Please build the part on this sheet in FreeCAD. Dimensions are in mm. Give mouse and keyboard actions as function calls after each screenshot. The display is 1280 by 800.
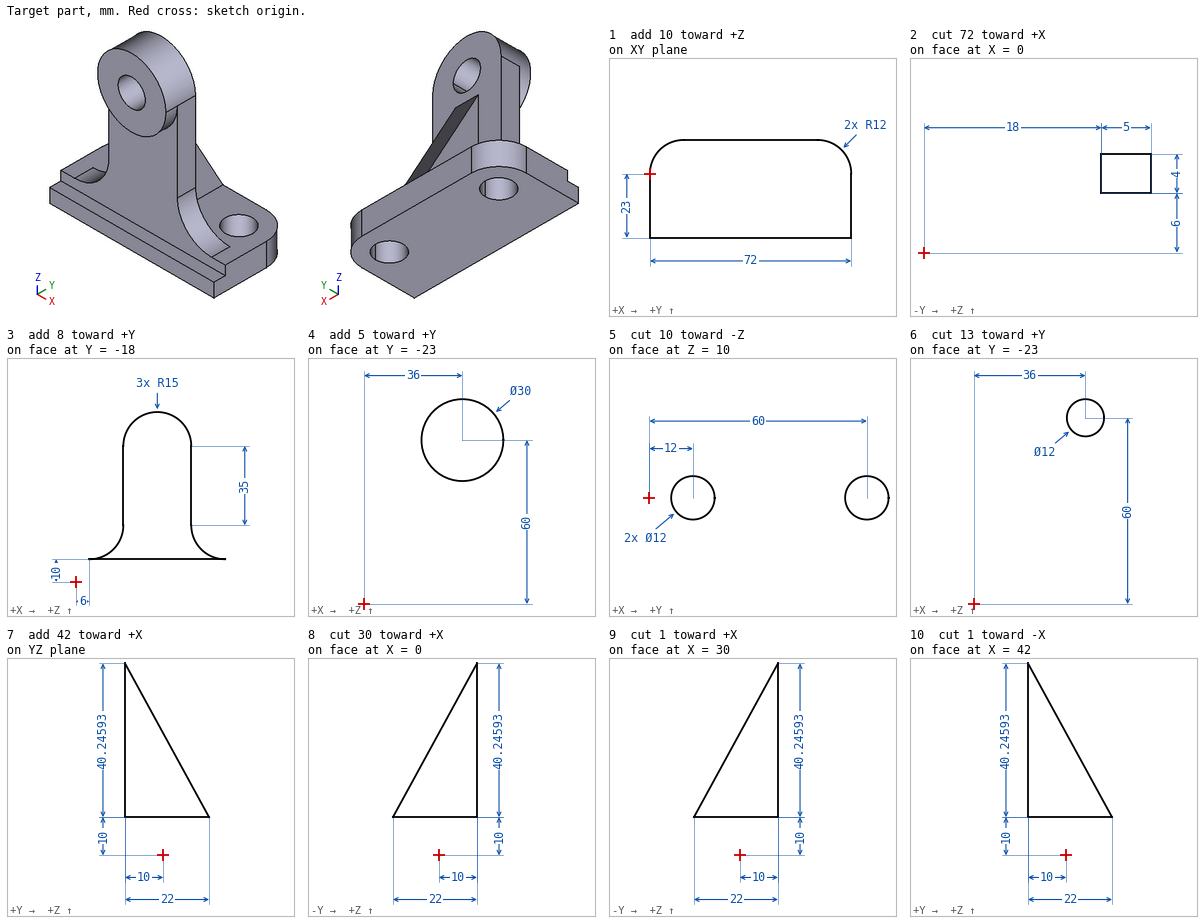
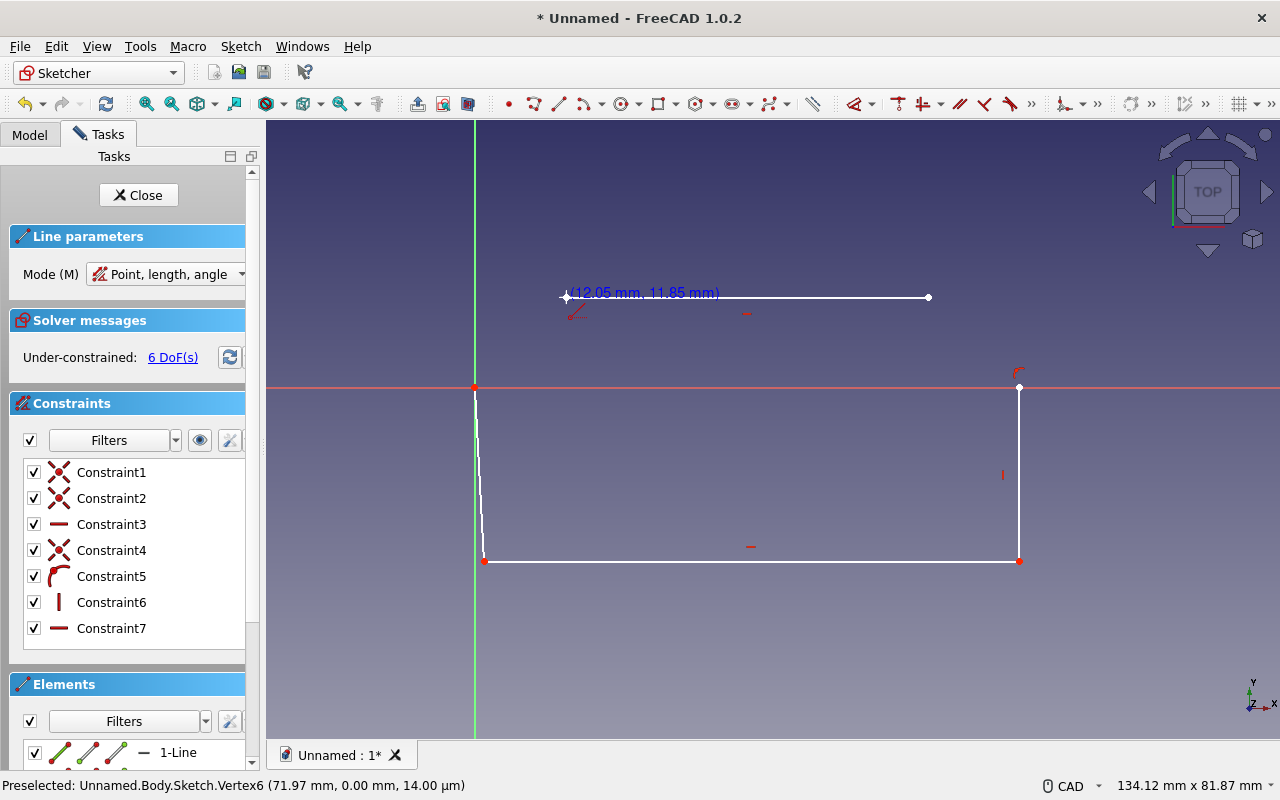
key(g)
key(3)
key(a)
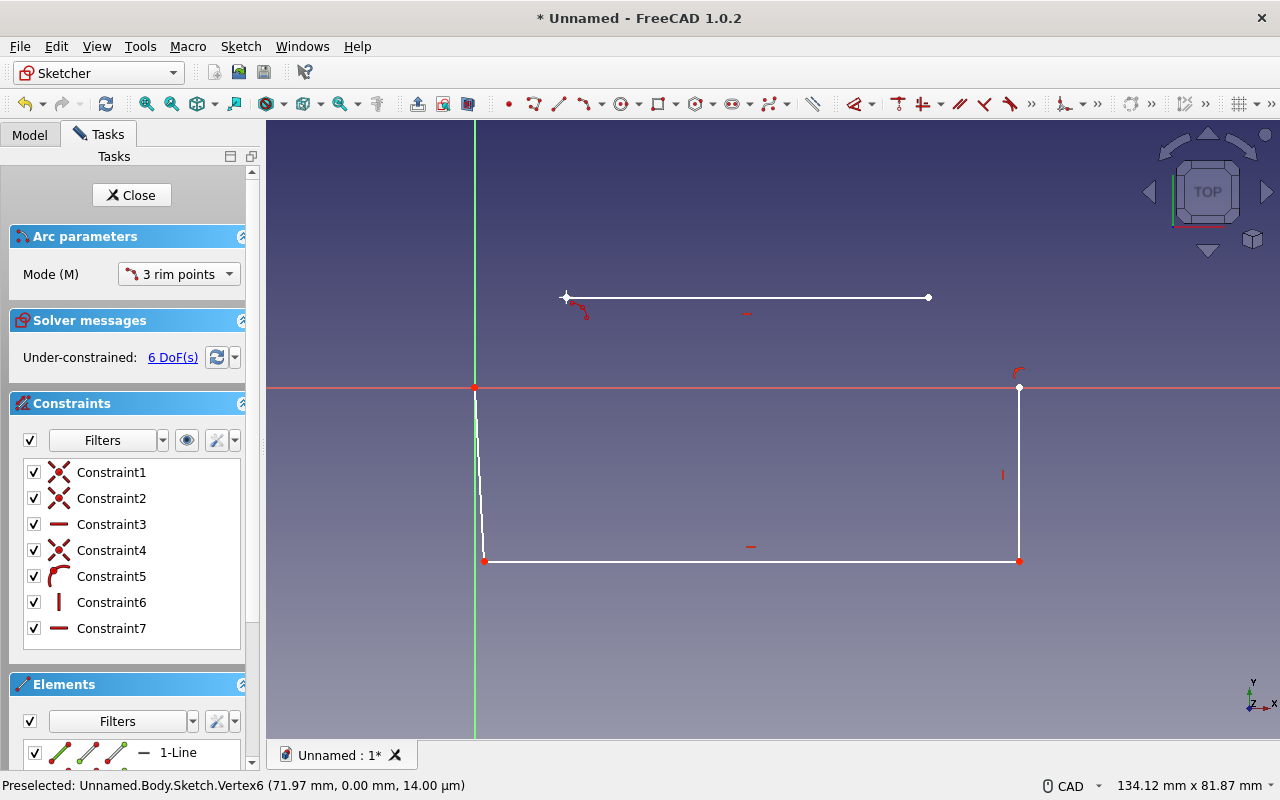
click(1019, 388)
click(928, 298)
click(993, 323)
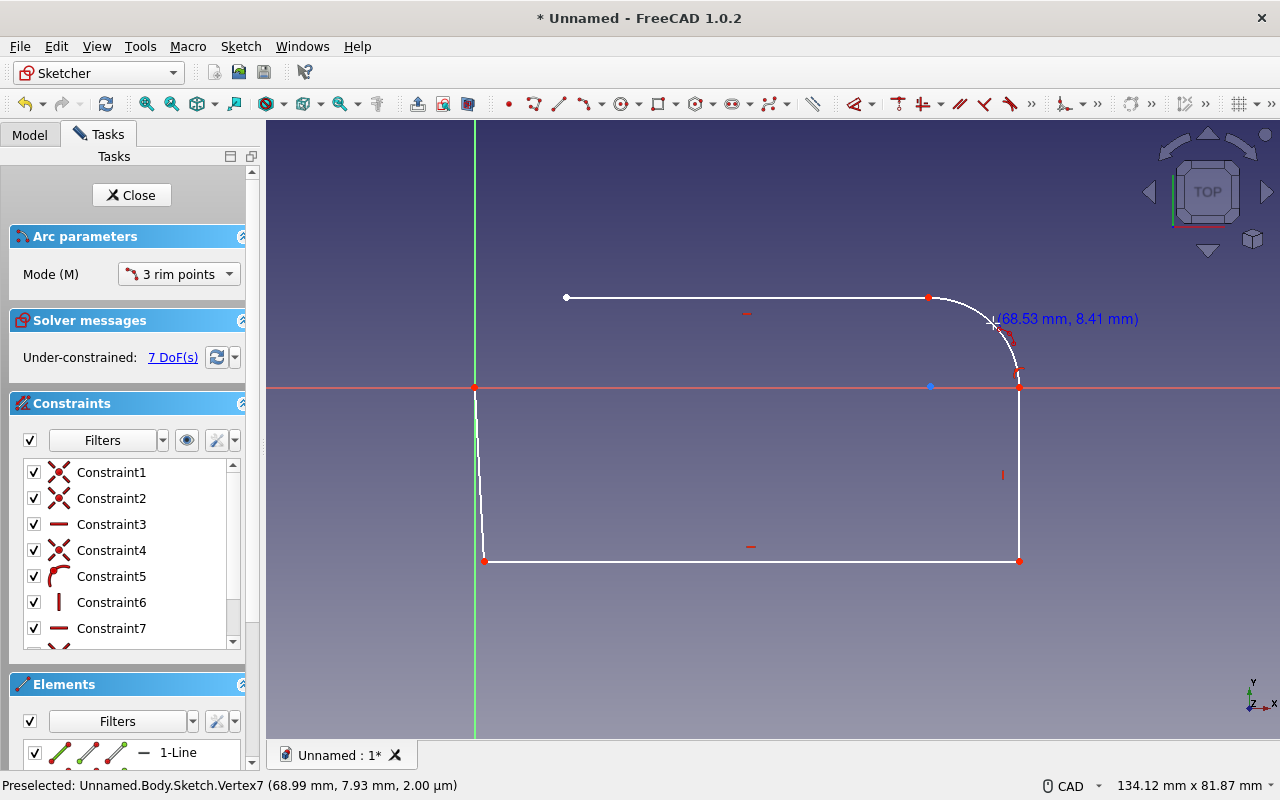
click(566, 298)
click(475, 388)
click(501, 323)
key(Escape)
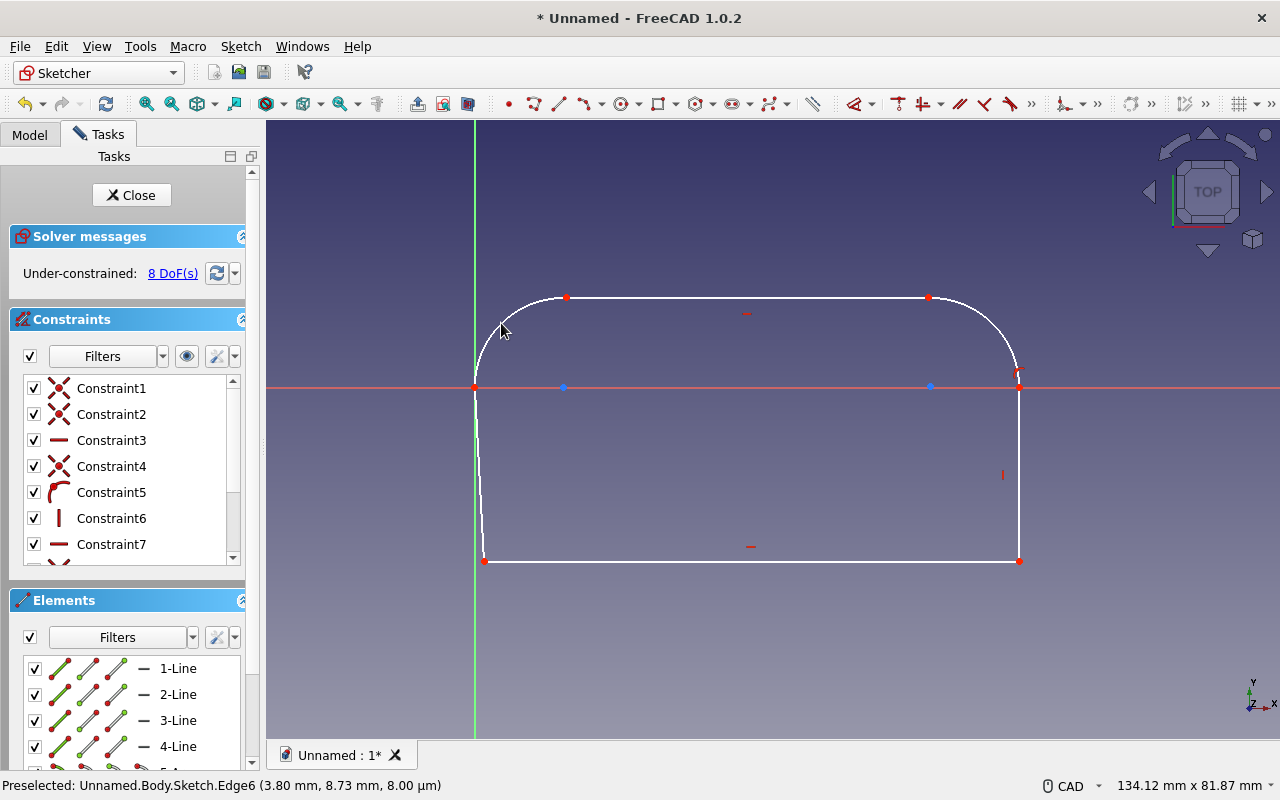
click(478, 440)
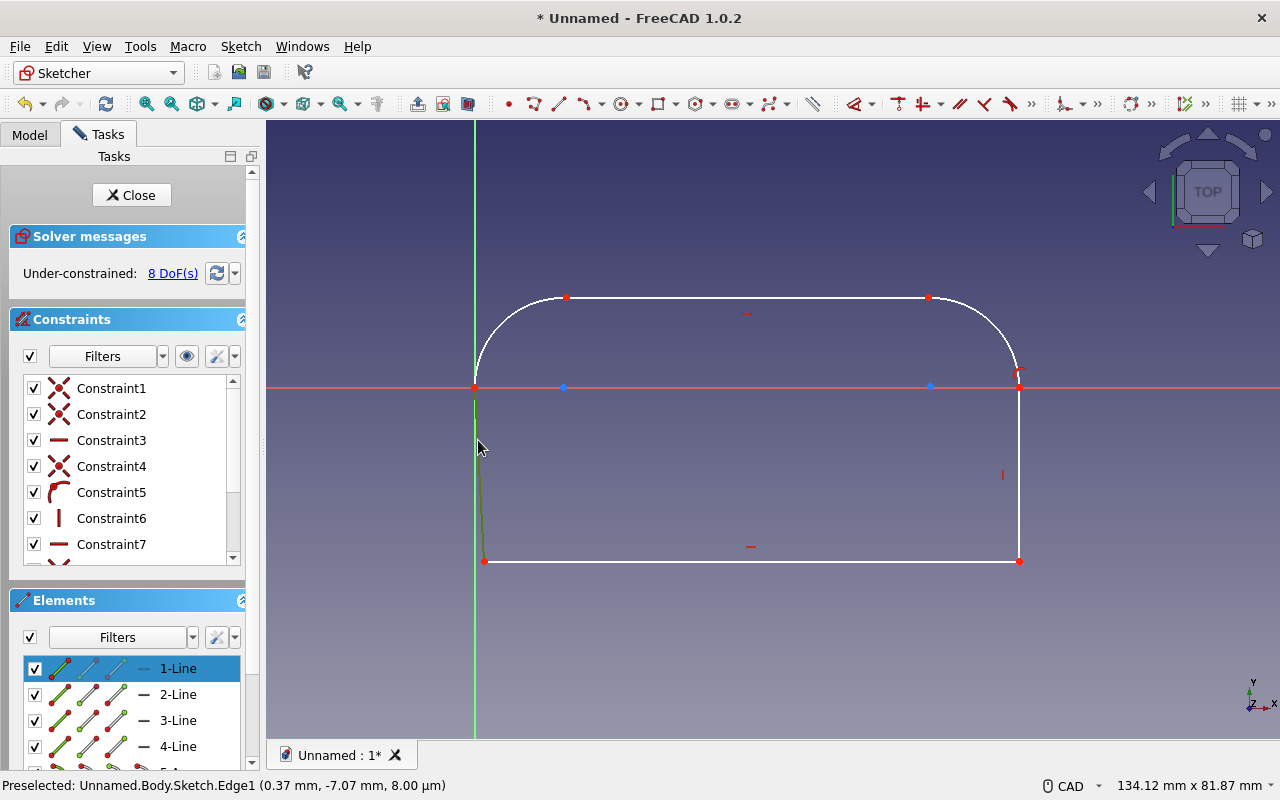
click(525, 307)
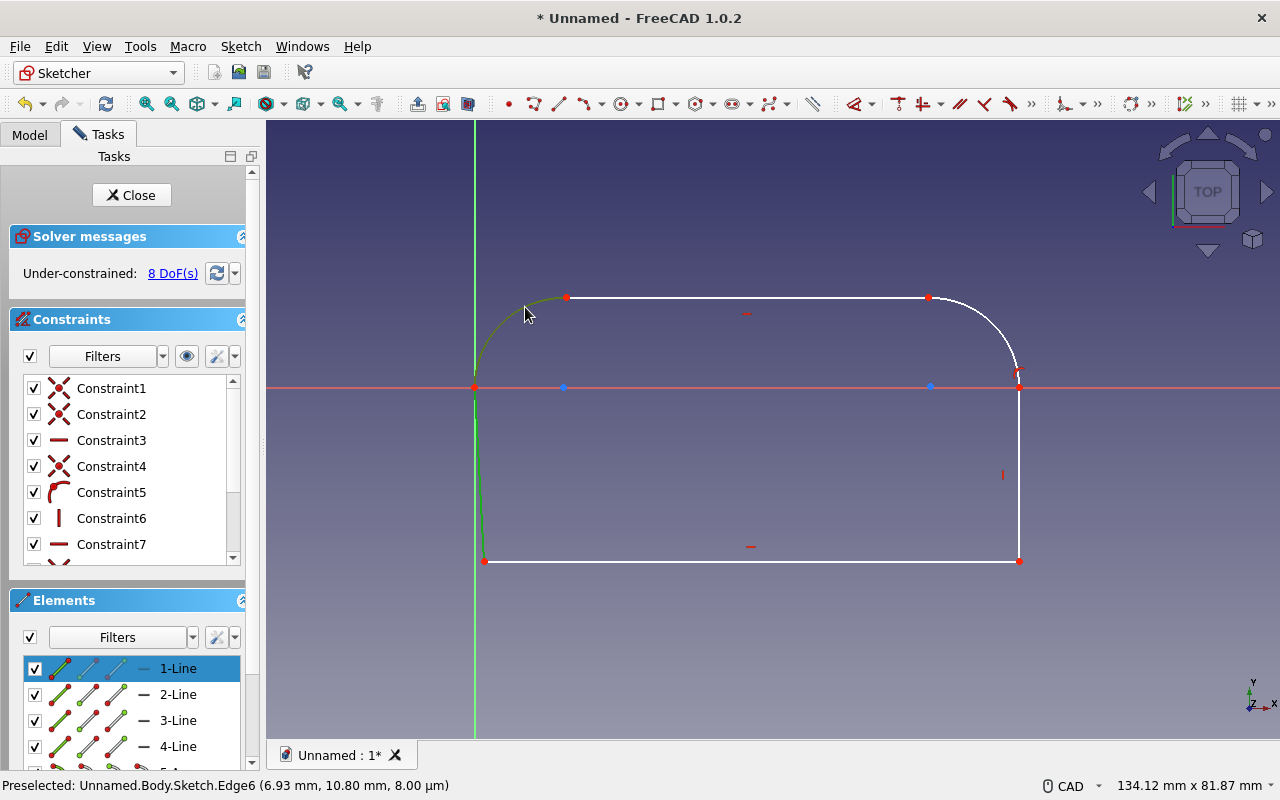
click(1010, 104)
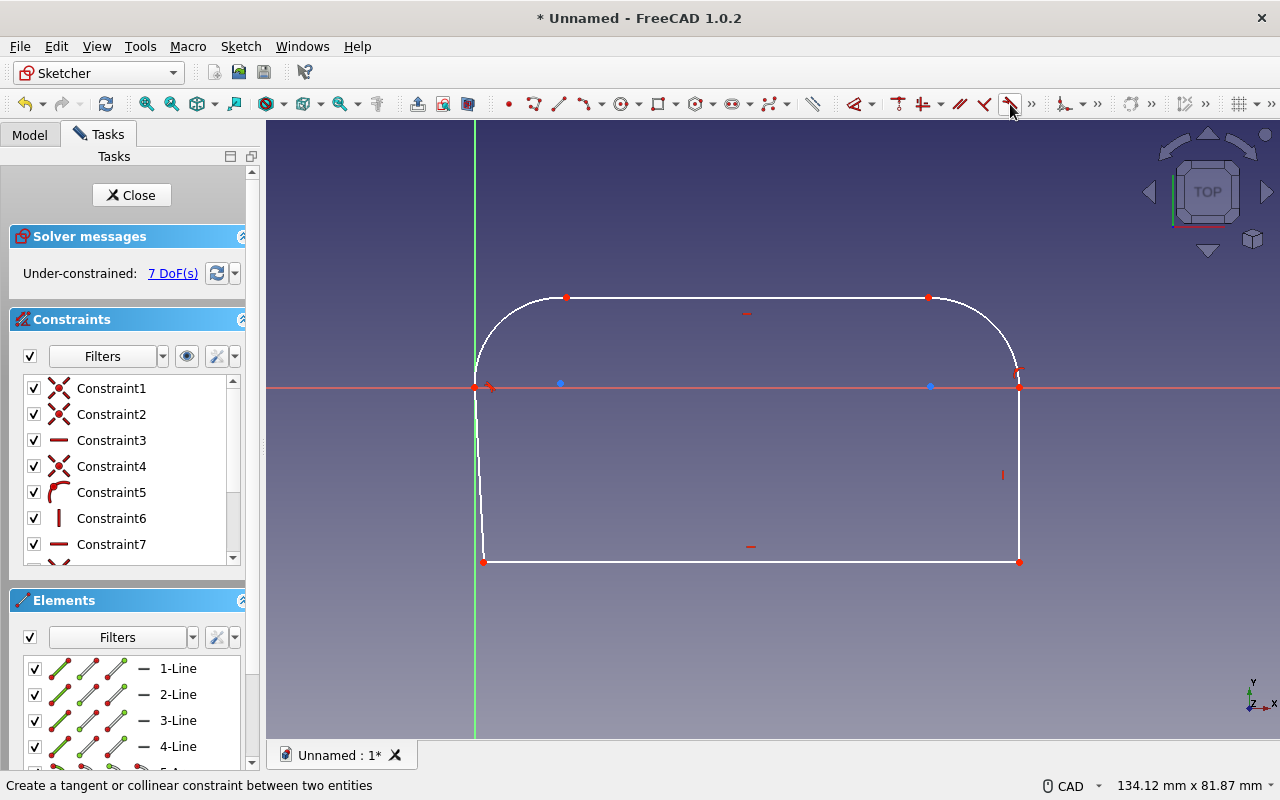
click(1019, 510)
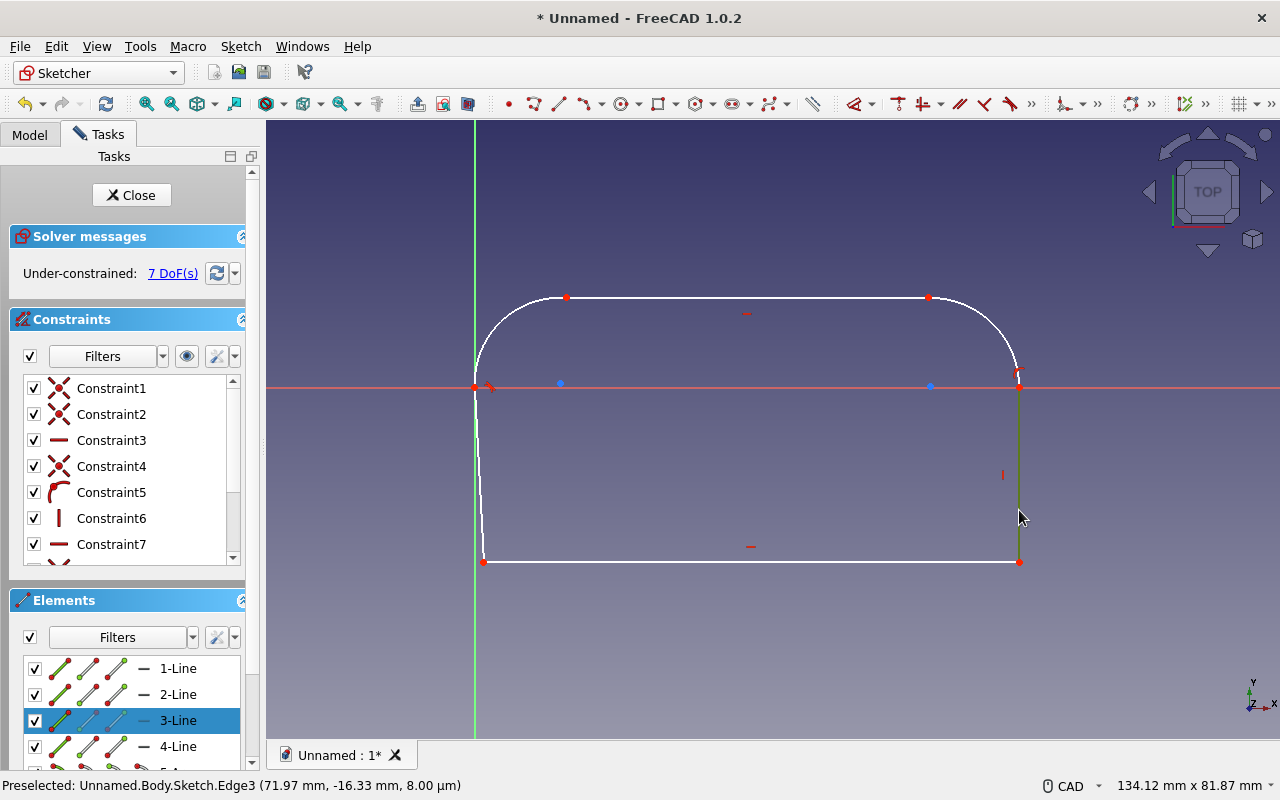
click(1009, 346)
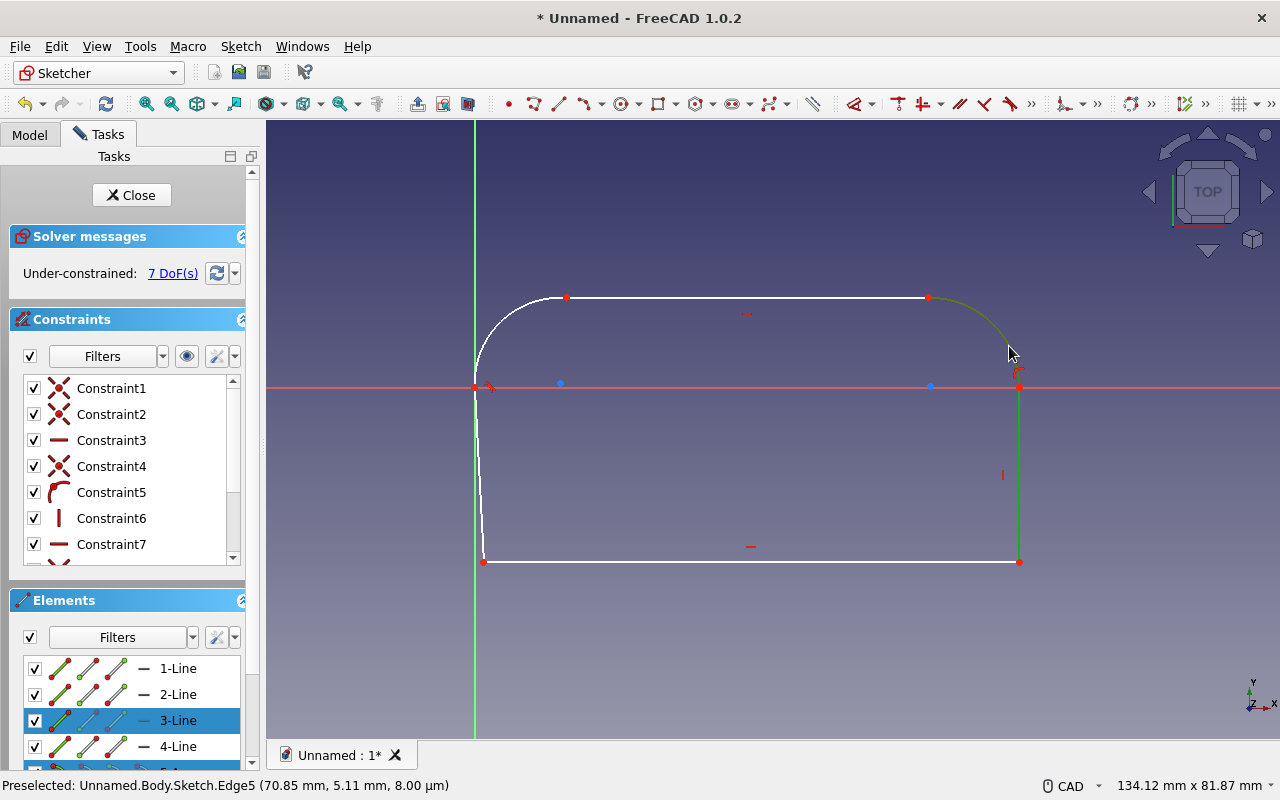
click(1010, 104)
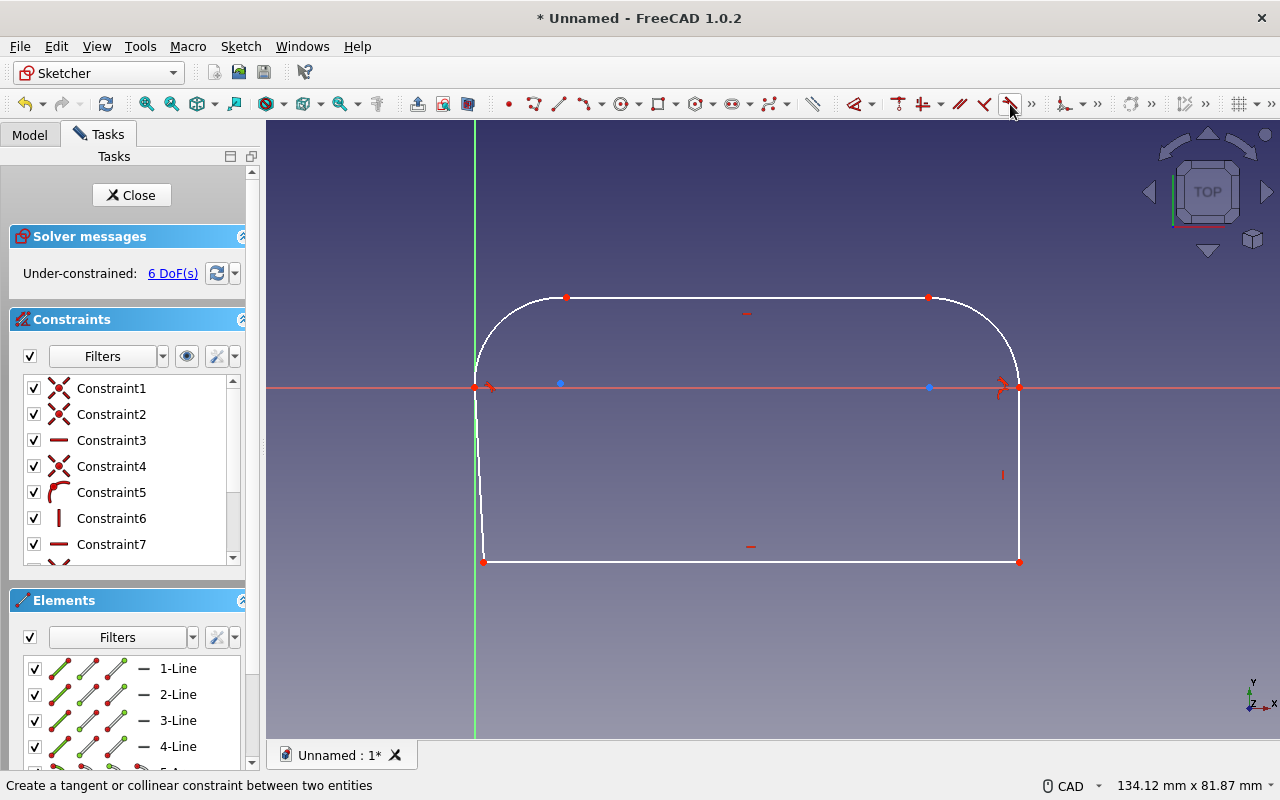
click(819, 298)